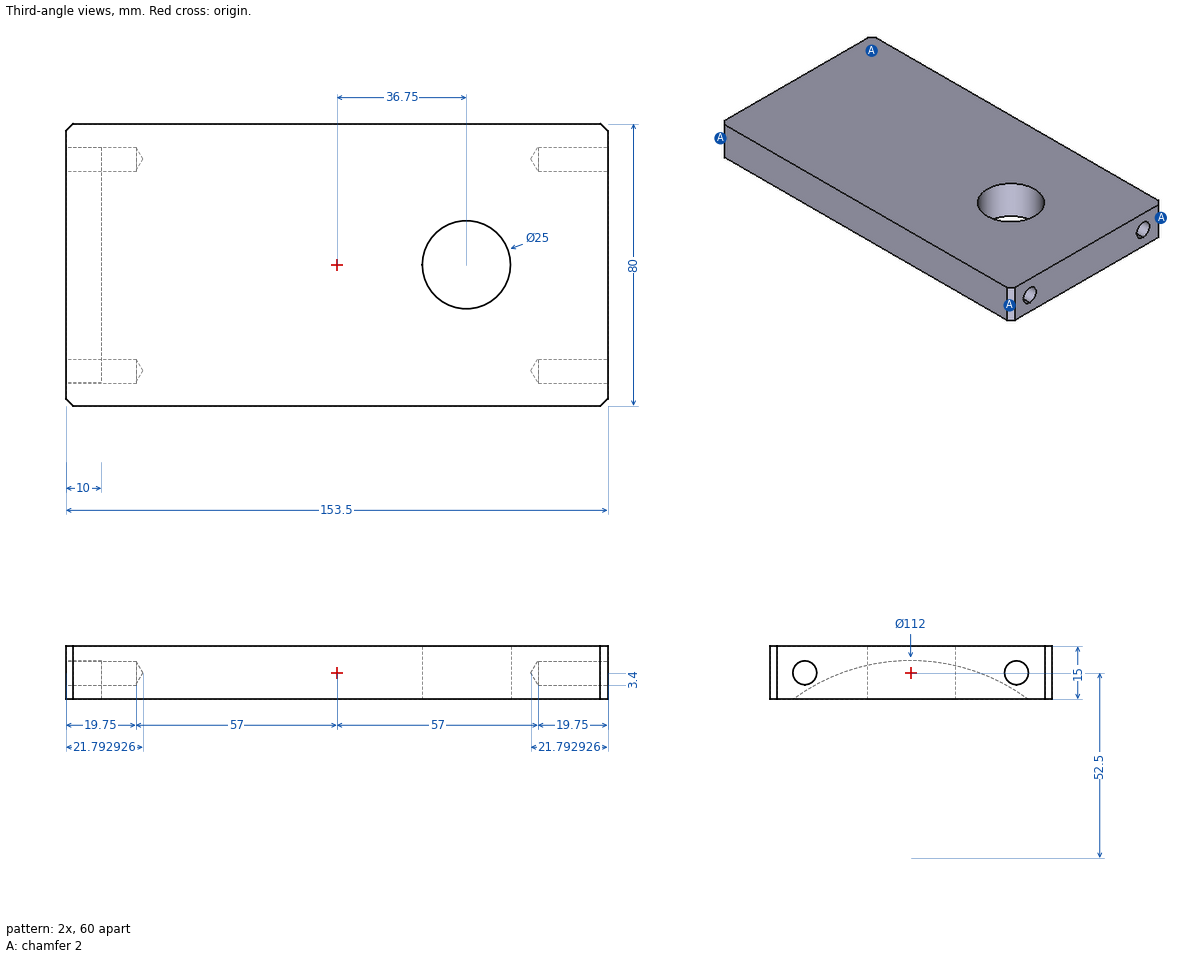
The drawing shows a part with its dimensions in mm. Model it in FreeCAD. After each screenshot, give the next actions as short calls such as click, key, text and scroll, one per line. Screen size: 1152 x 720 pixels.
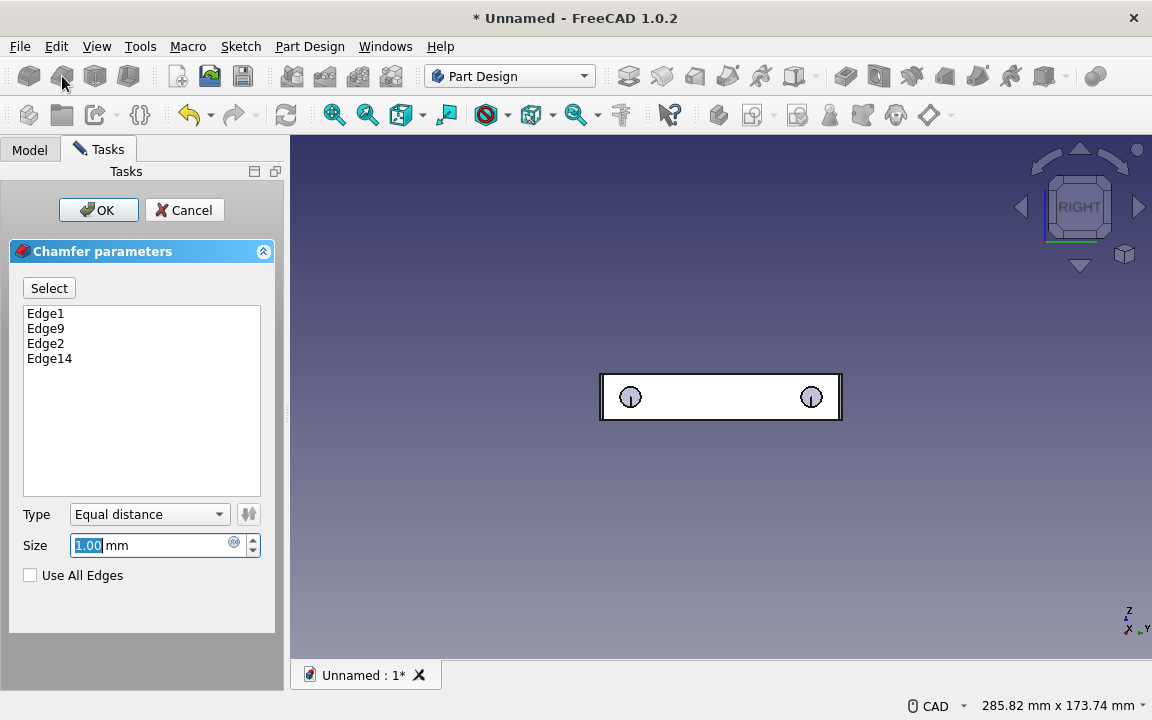
text(2)
key(Tab)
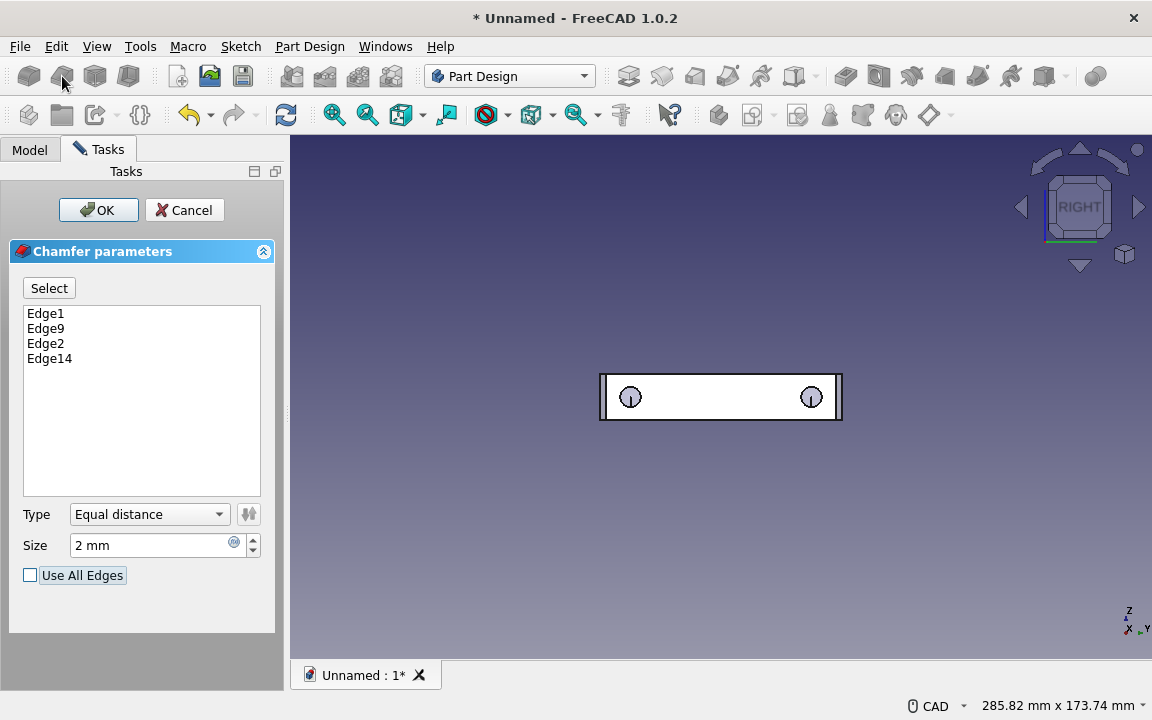
click(99, 210)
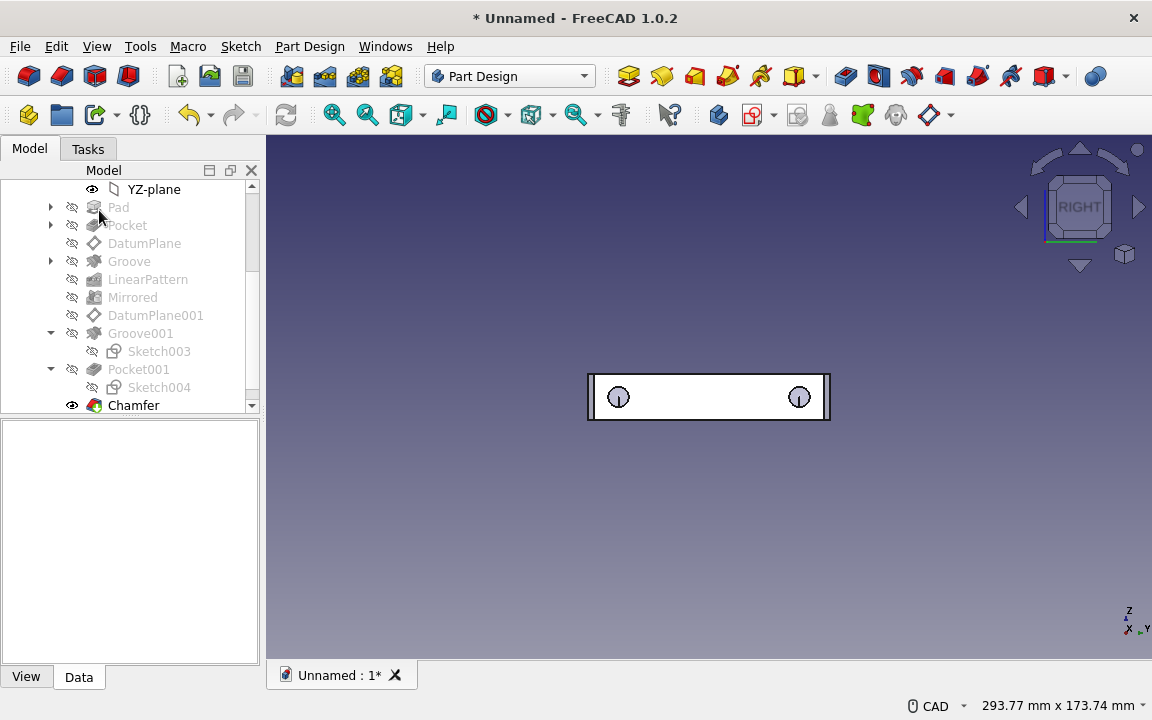
key(0)